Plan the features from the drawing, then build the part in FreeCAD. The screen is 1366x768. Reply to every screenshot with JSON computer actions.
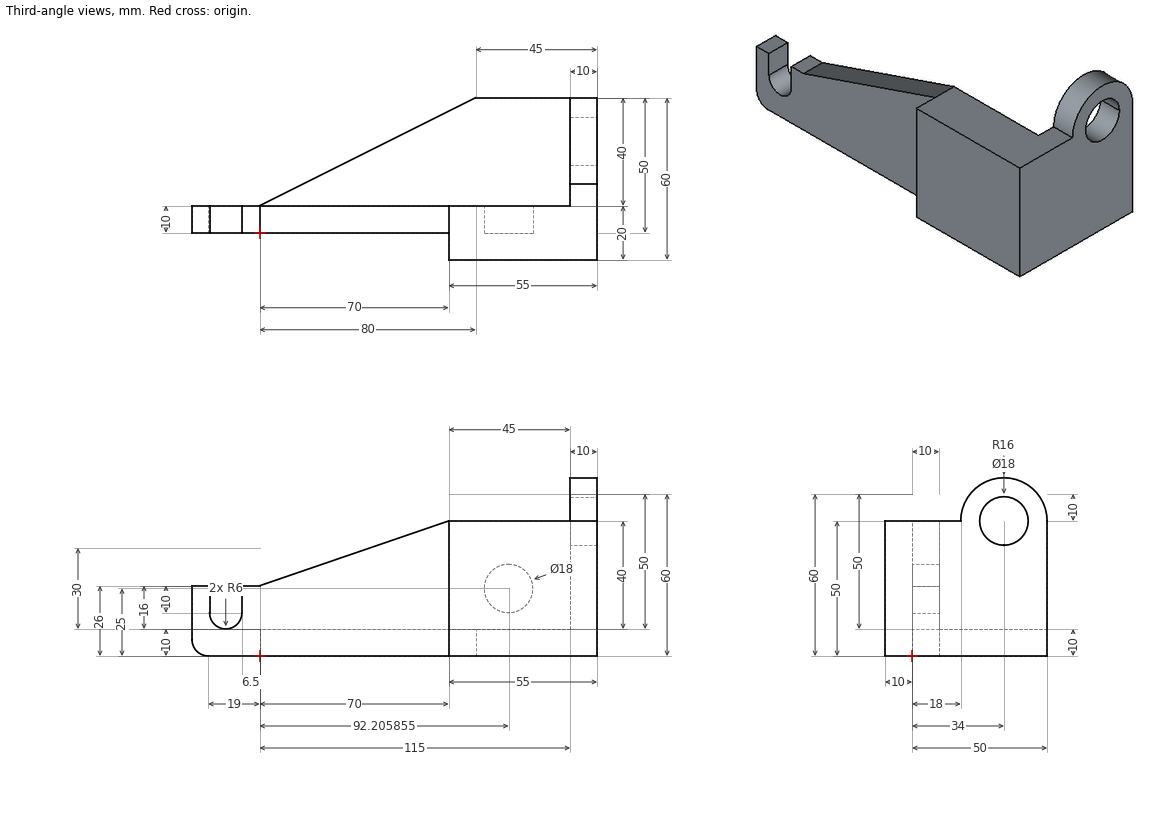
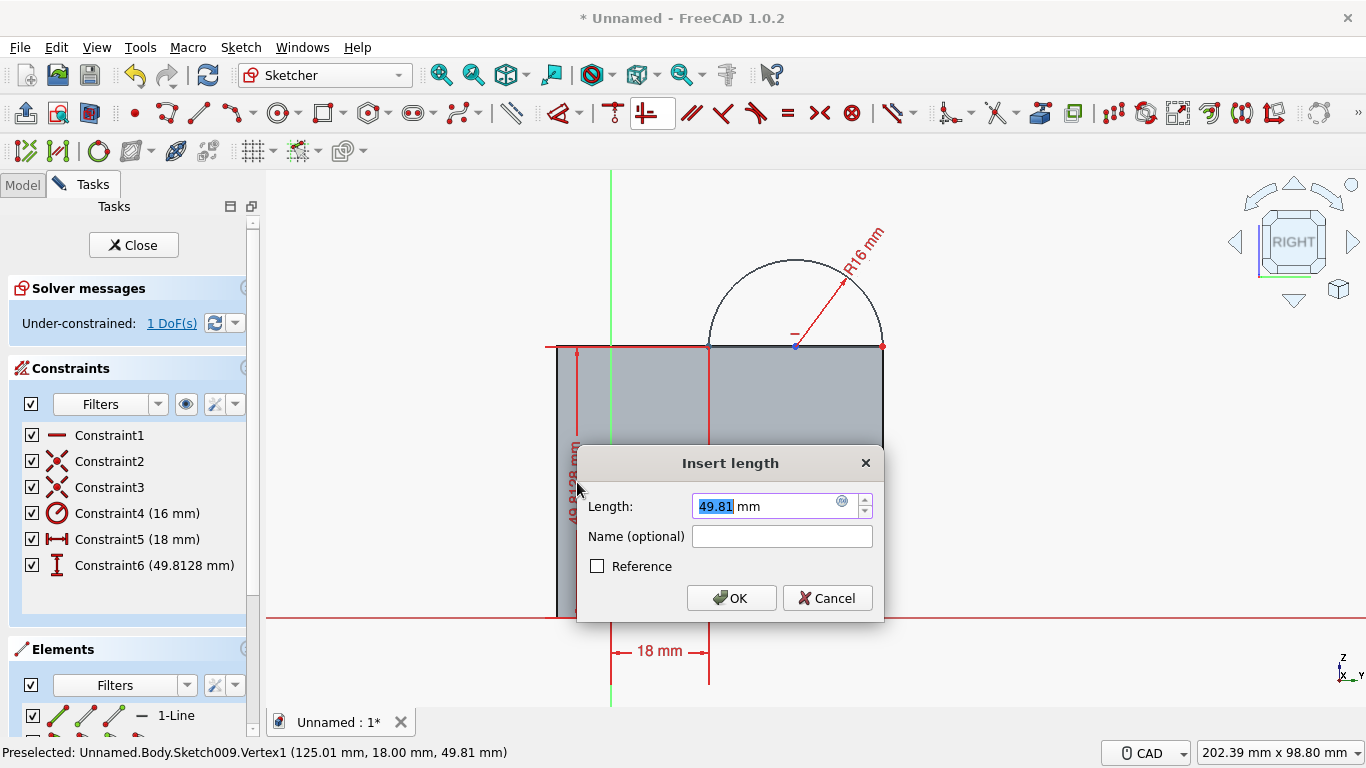
{"action": "type", "text": "50"}
{"action": "key", "text": "Return"}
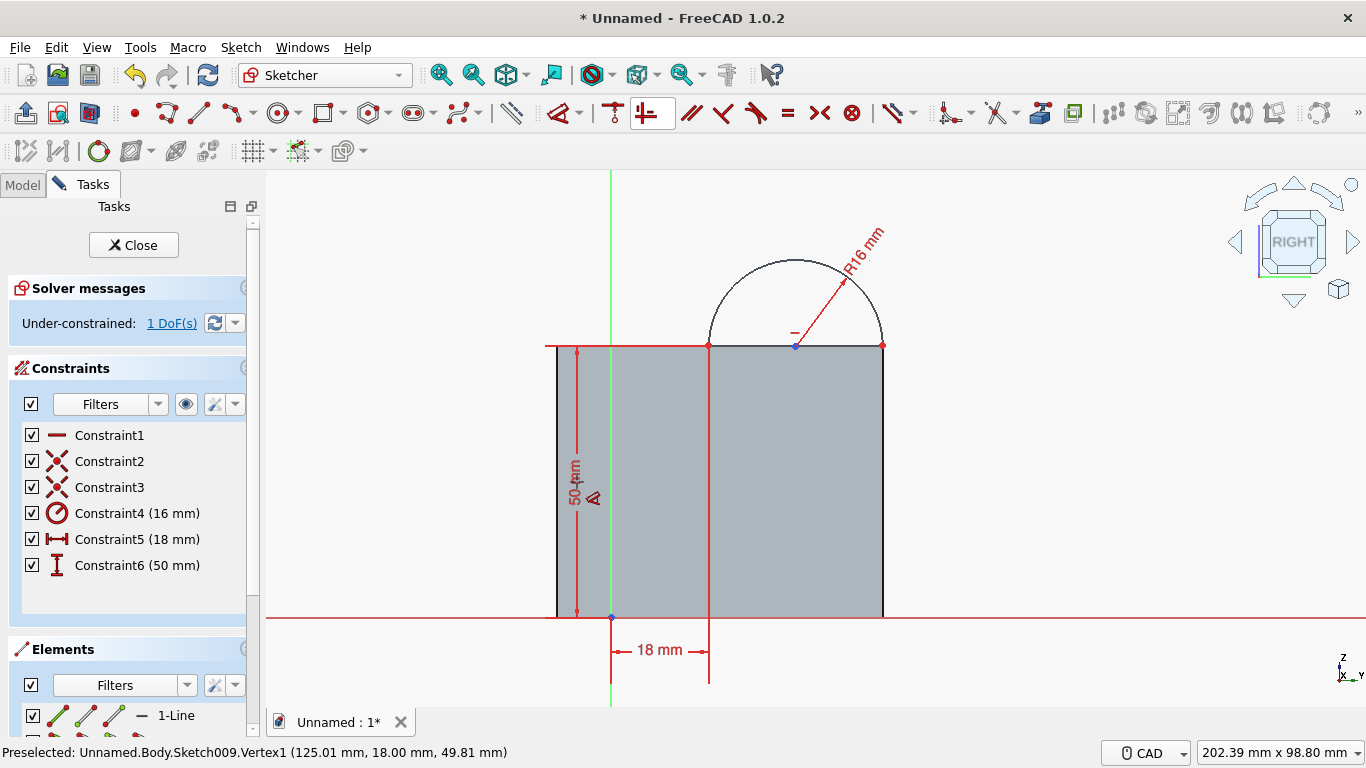
{"action": "left_click", "coordinate": [796, 347]}
{"action": "left_click", "coordinate": [577, 420]}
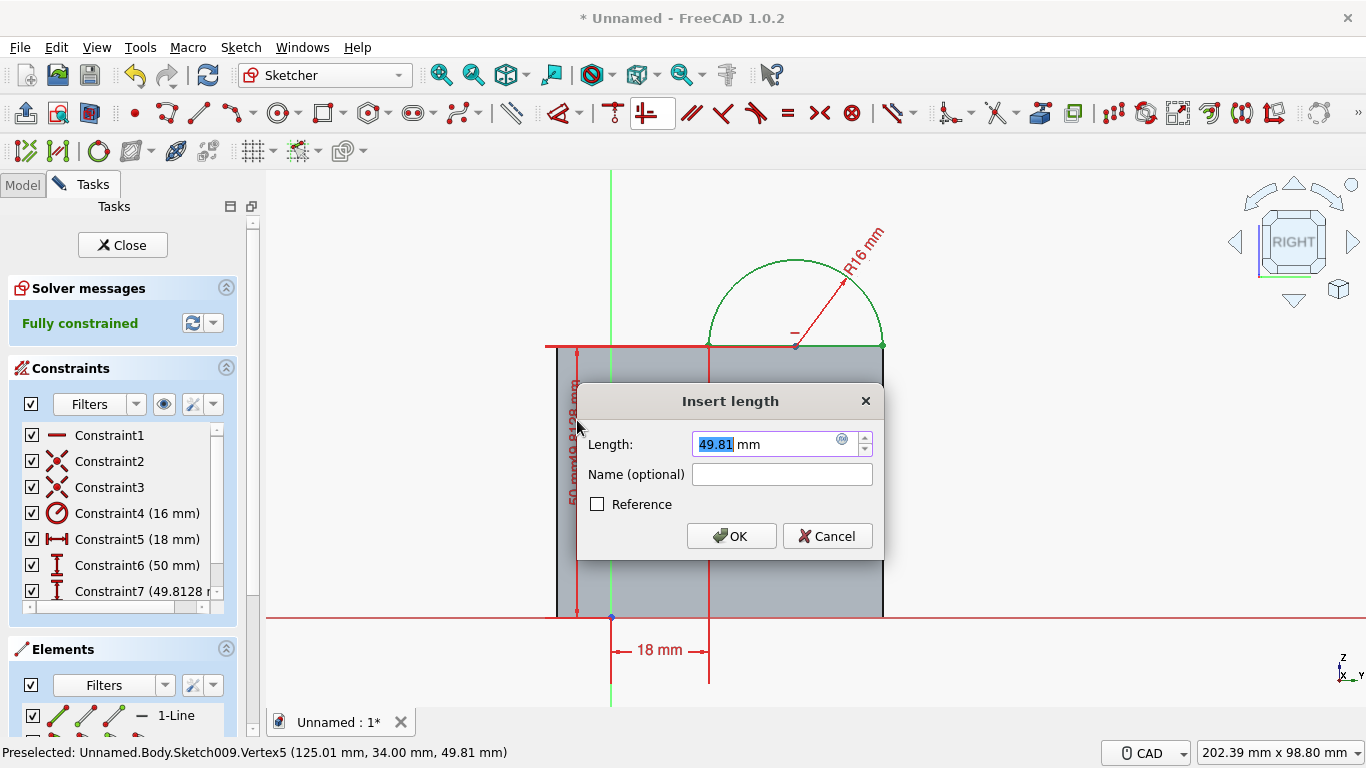
{"action": "type", "text": "50"}
{"action": "key", "text": "Return"}
{"action": "key", "text": "Escape"}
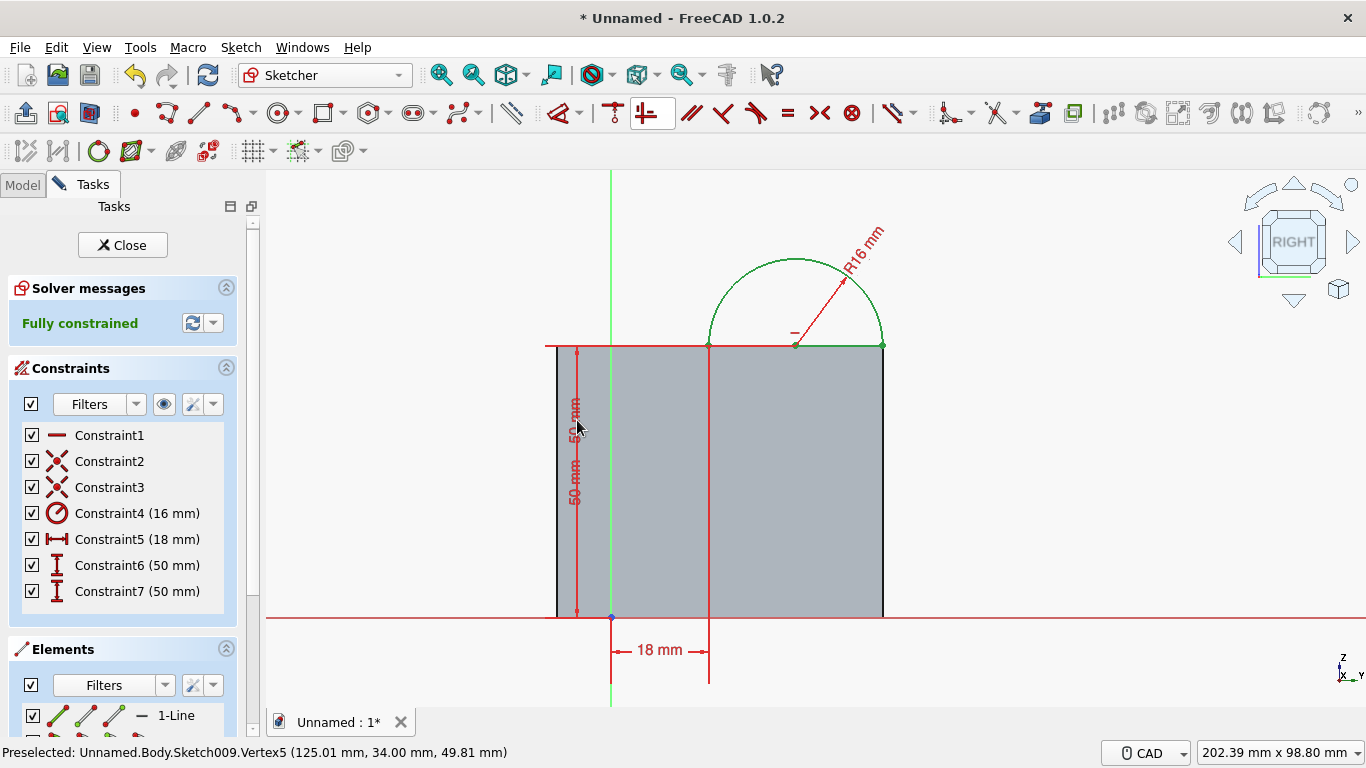
{"action": "left_click", "coordinate": [123, 245]}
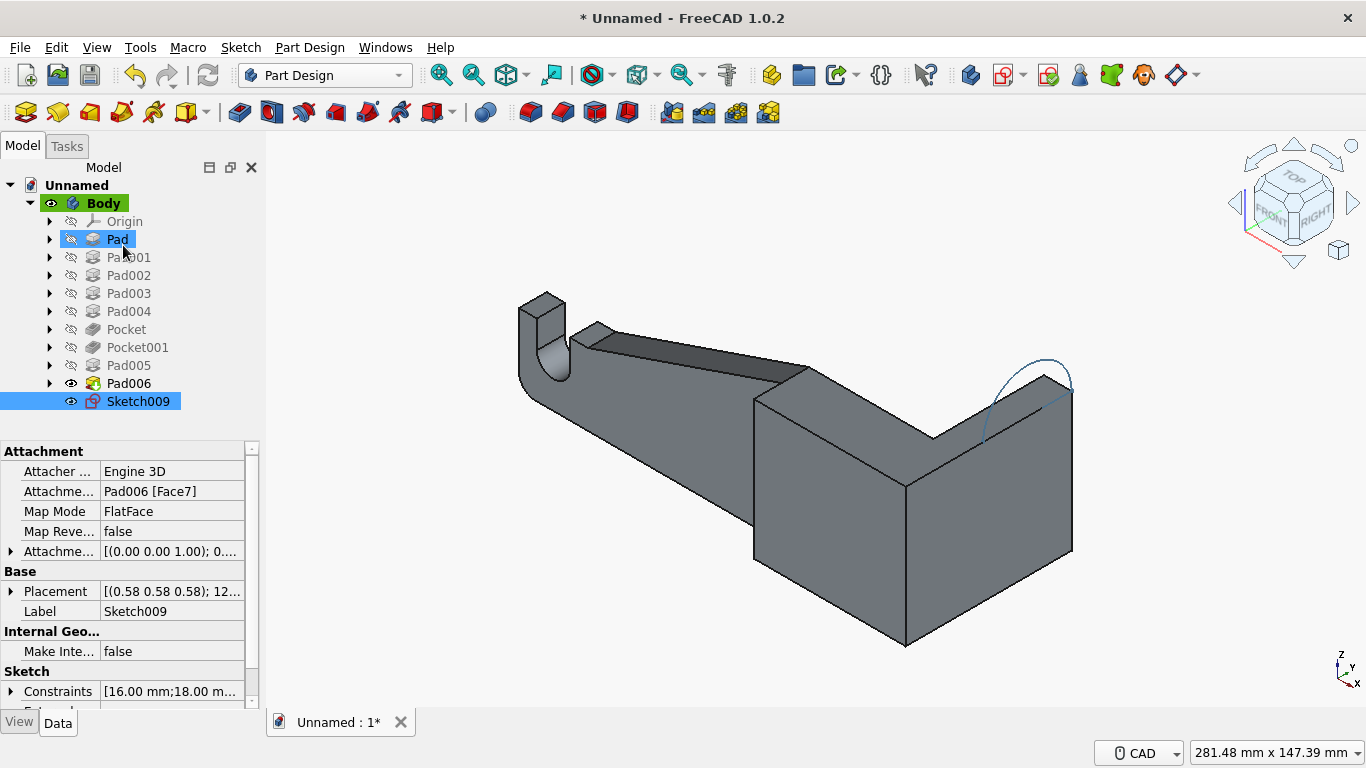
{"action": "left_click", "coordinate": [26, 112]}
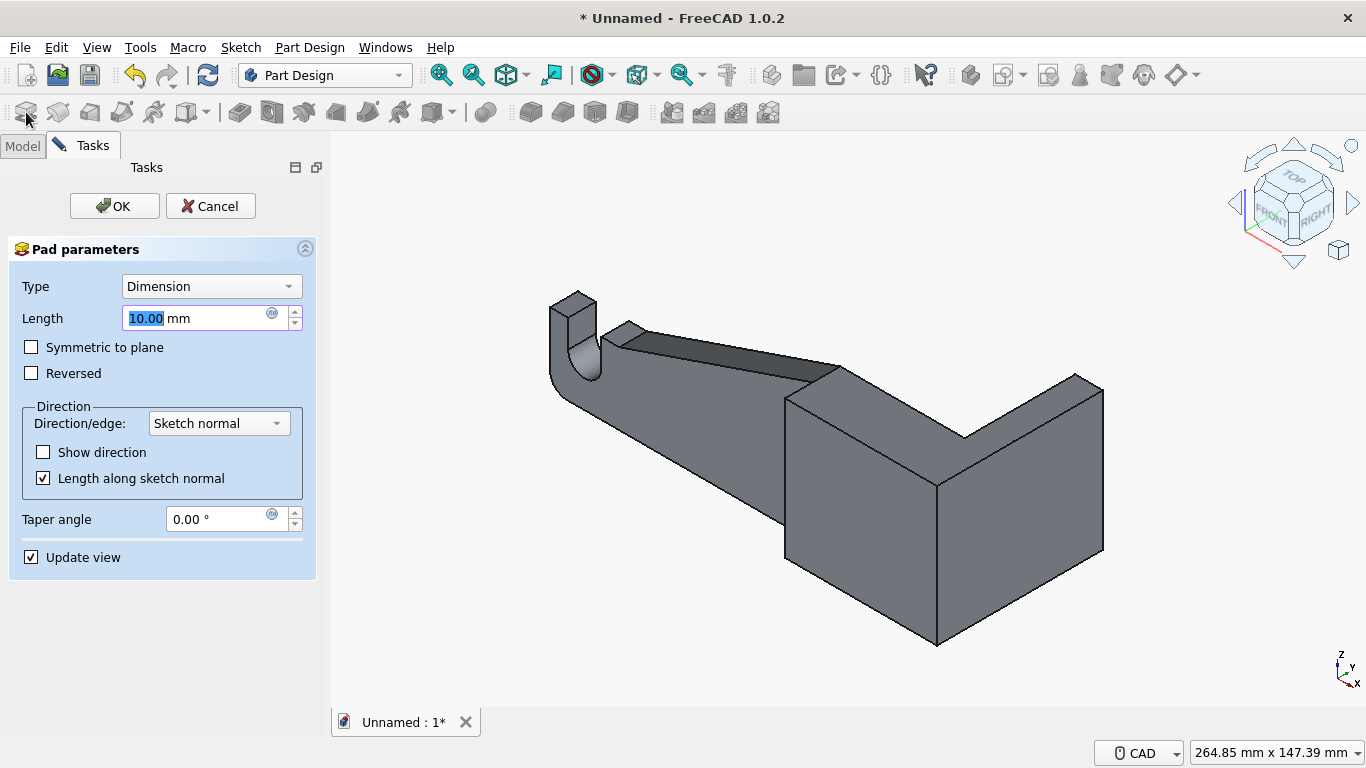
{"action": "type", "text": "10"}
{"action": "key", "text": "Tab"}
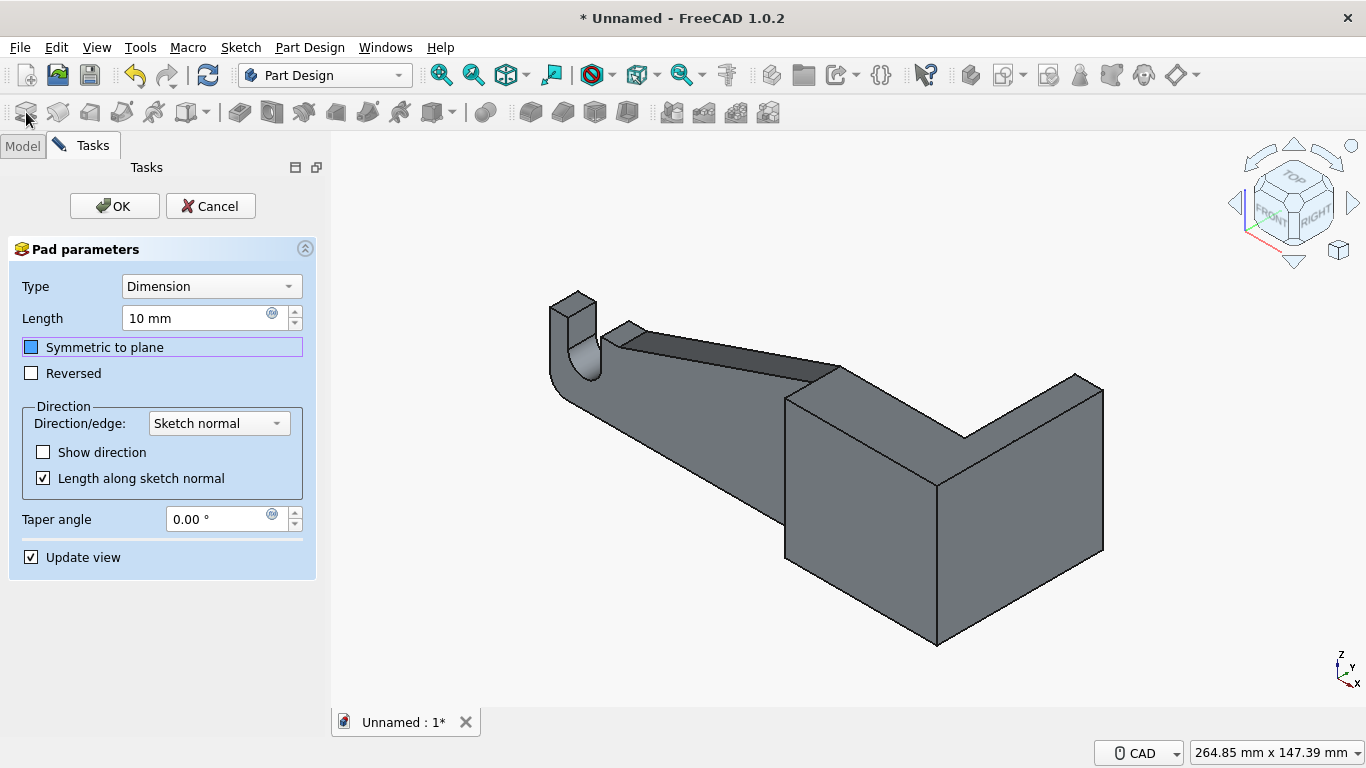
{"action": "left_click", "coordinate": [30, 373]}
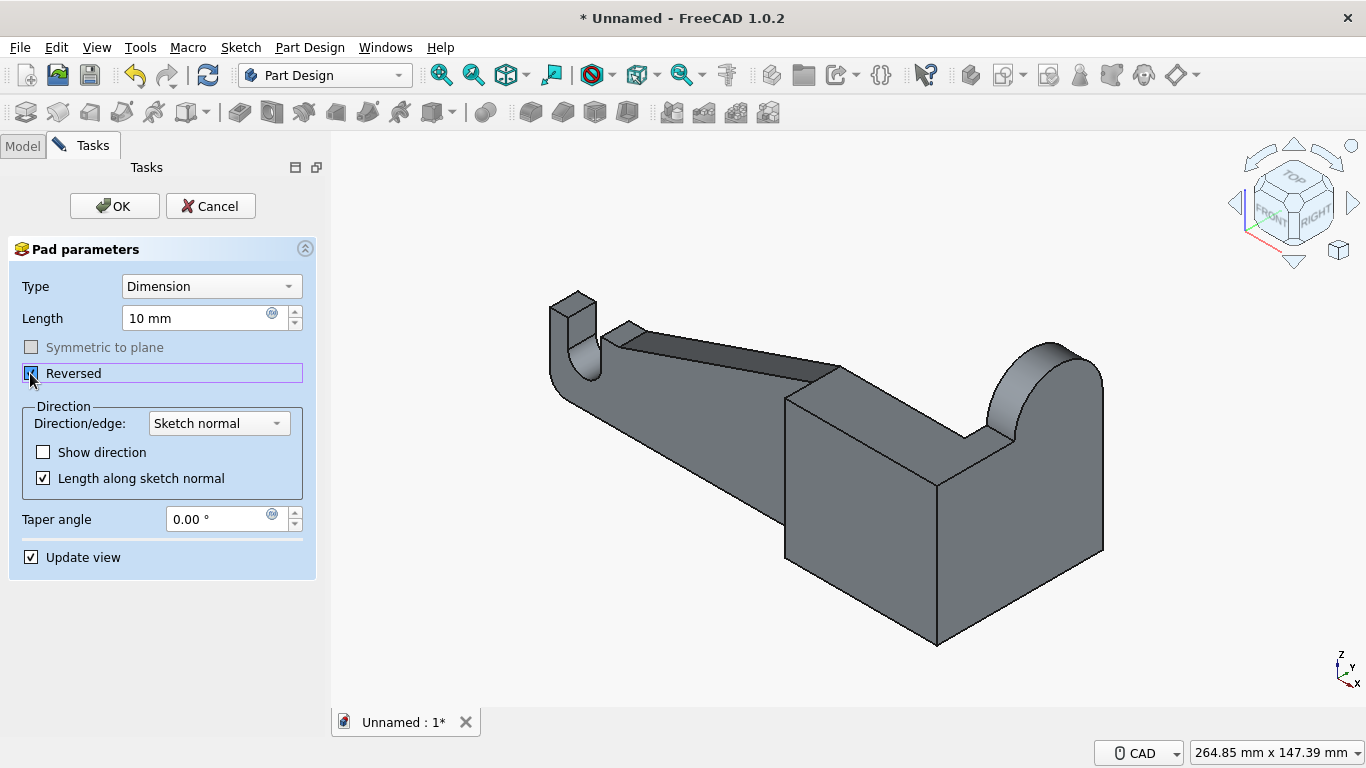
{"action": "left_click", "coordinate": [115, 206]}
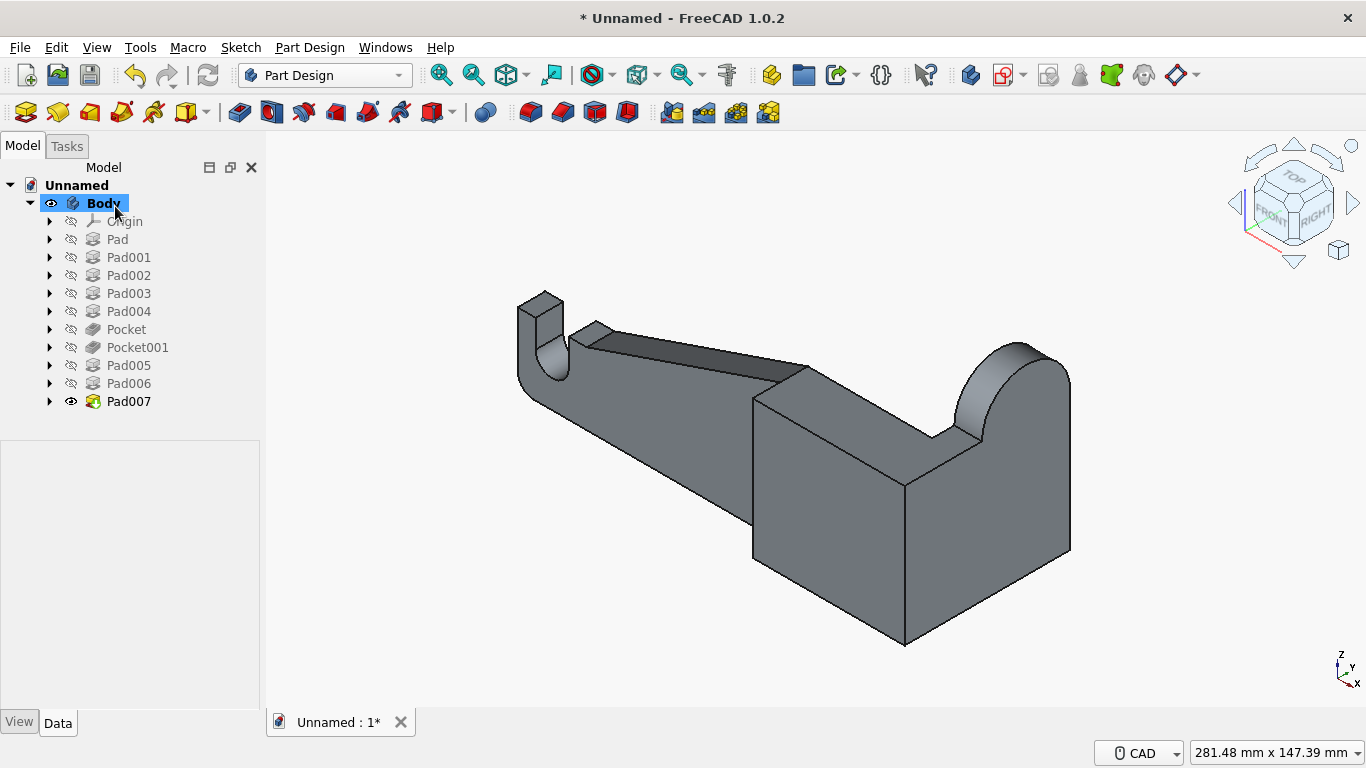
{"action": "left_click", "coordinate": [442, 76]}